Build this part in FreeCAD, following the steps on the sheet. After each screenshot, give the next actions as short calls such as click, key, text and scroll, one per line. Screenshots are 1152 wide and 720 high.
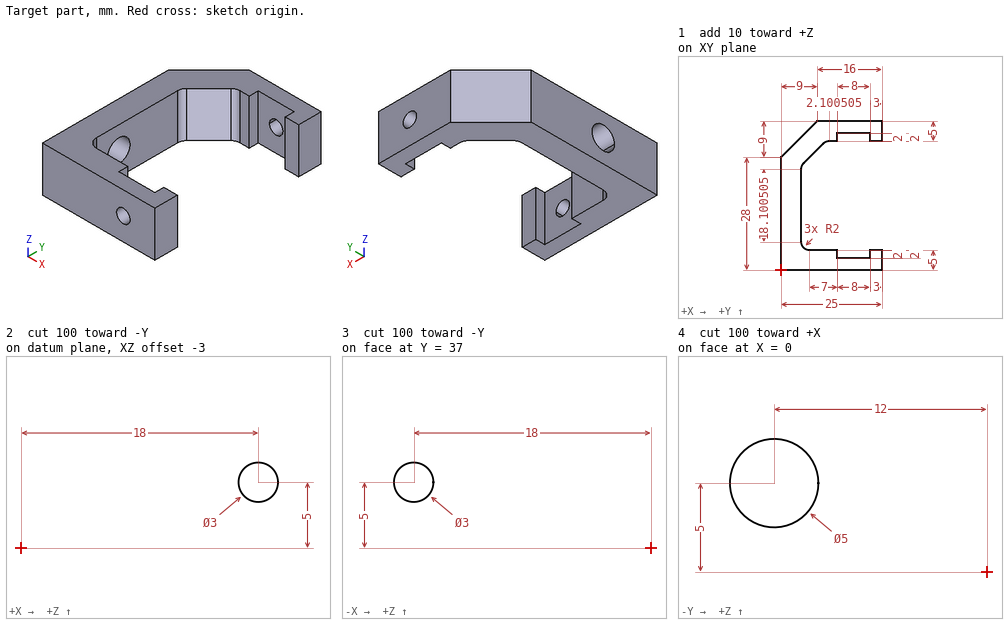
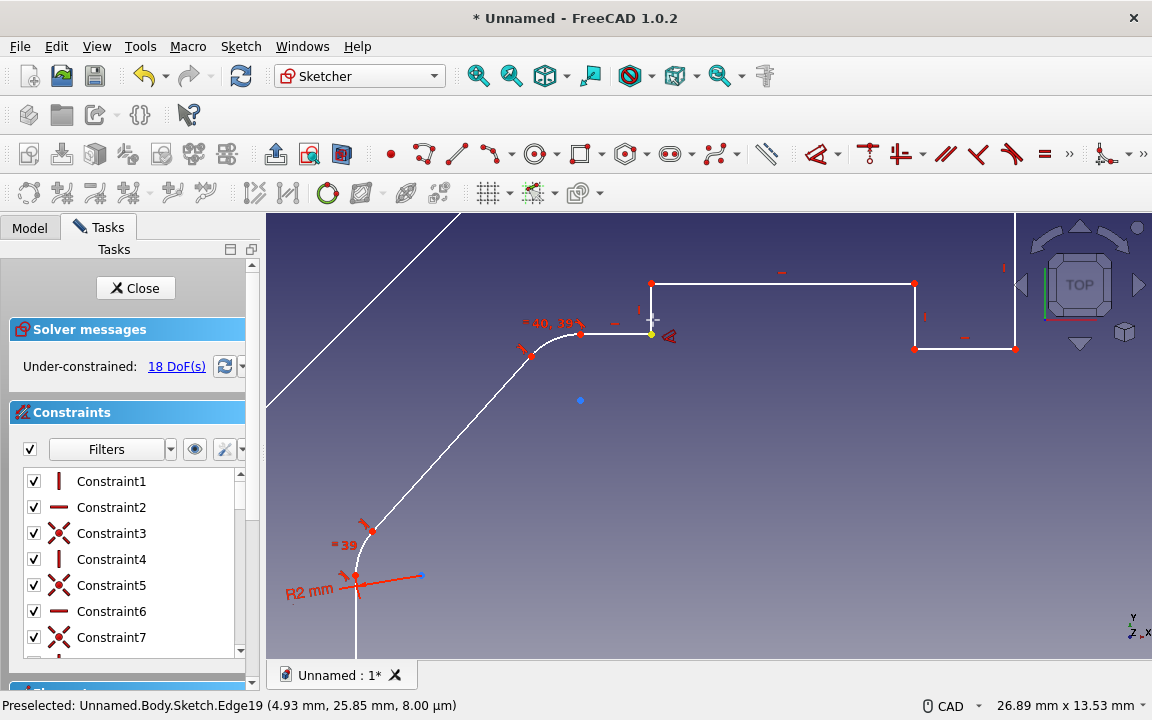
click(651, 319)
click(685, 309)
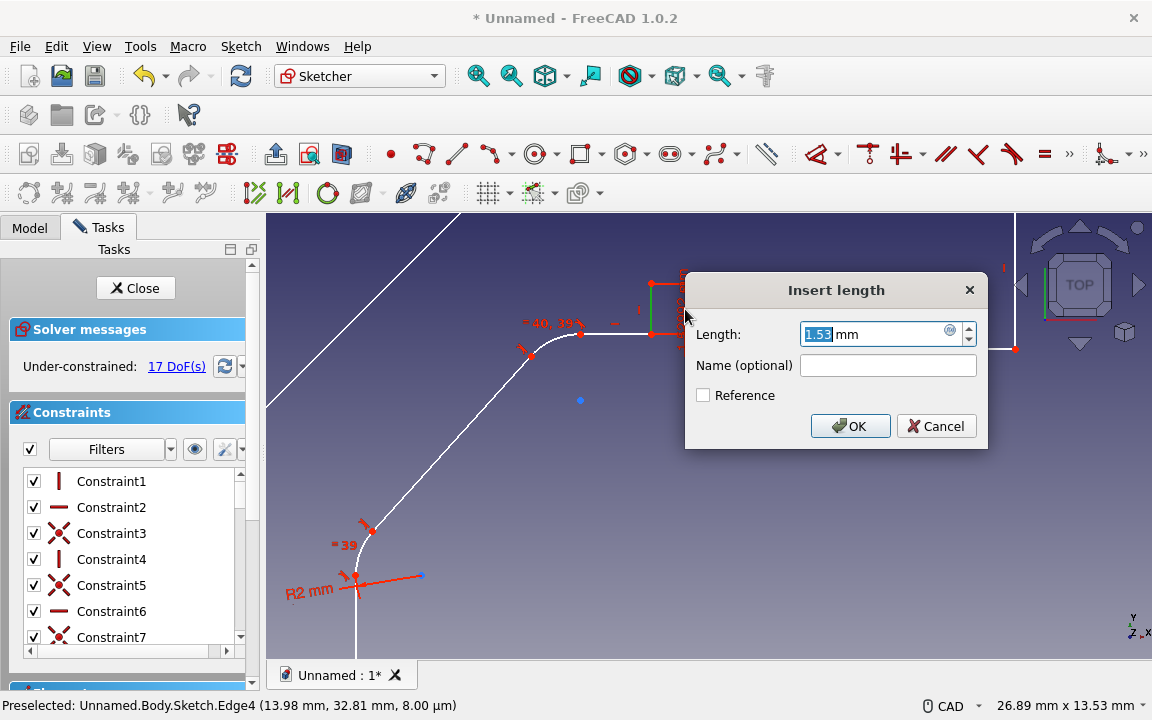
text(2)
key(Return)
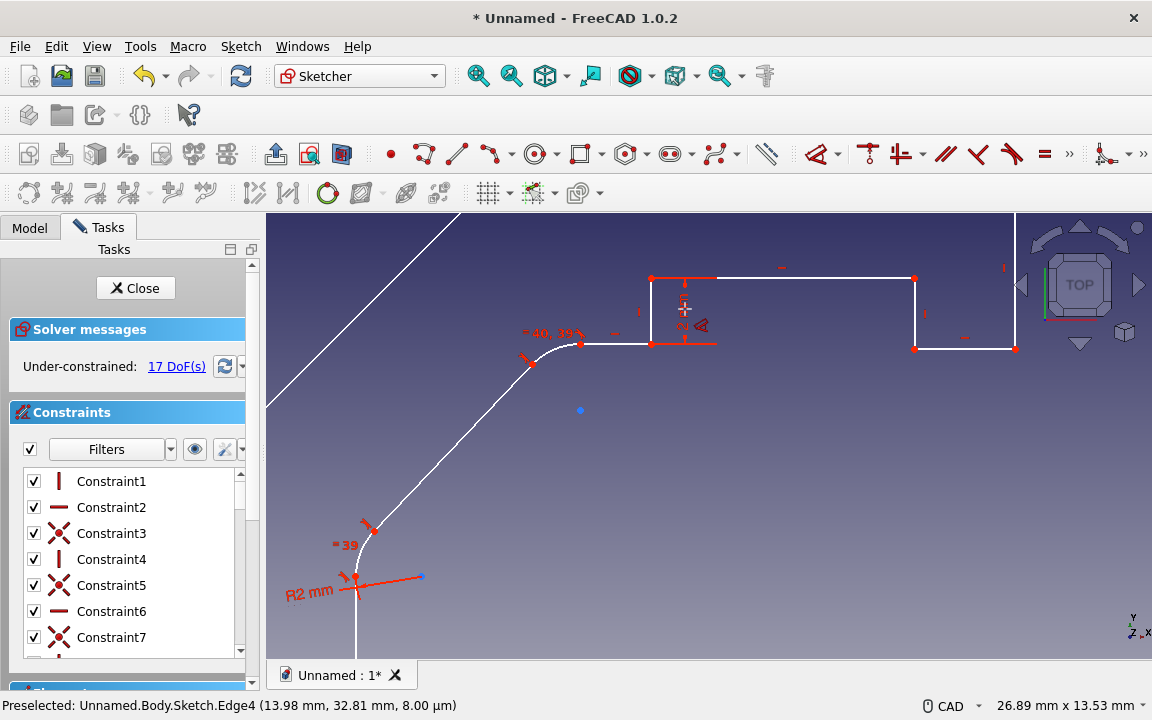
scroll(653, 320, down, 7)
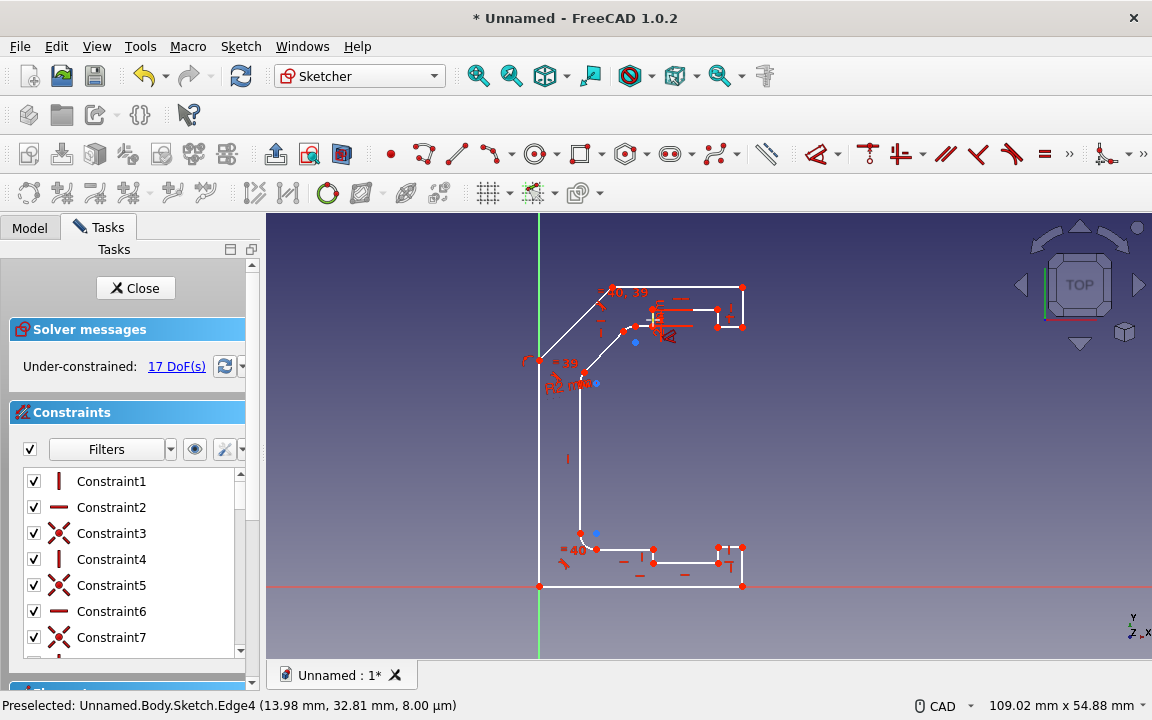
click(672, 310)
click(685, 344)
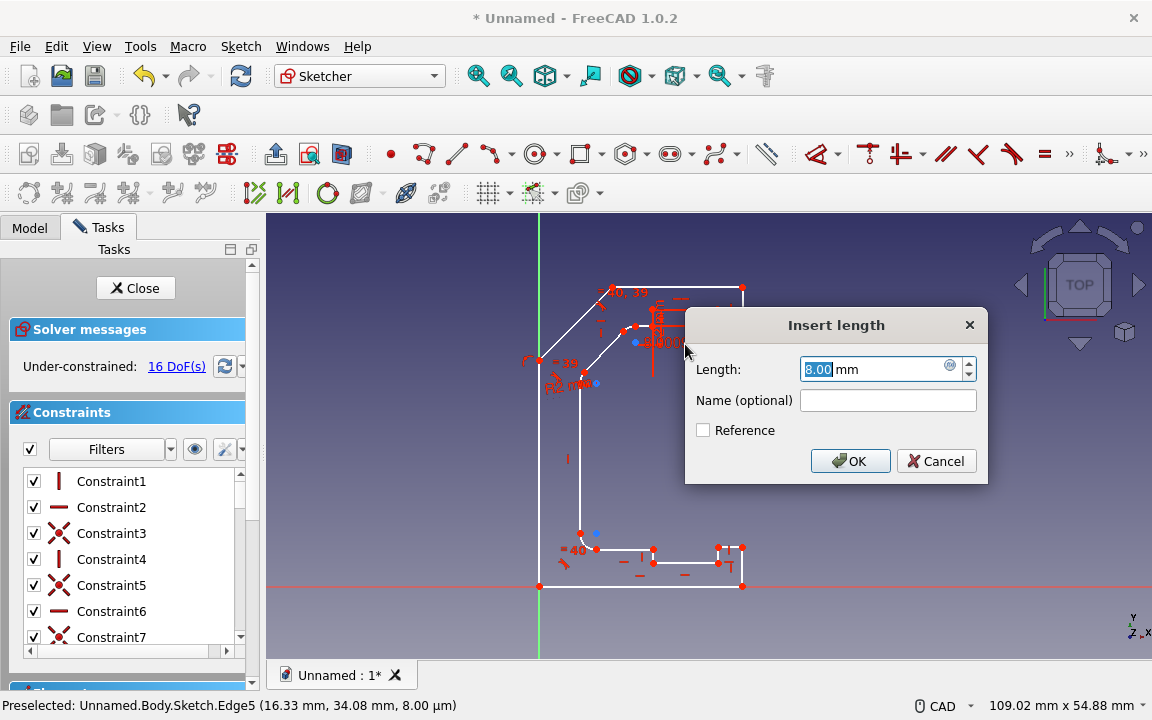
text(8)
key(Return)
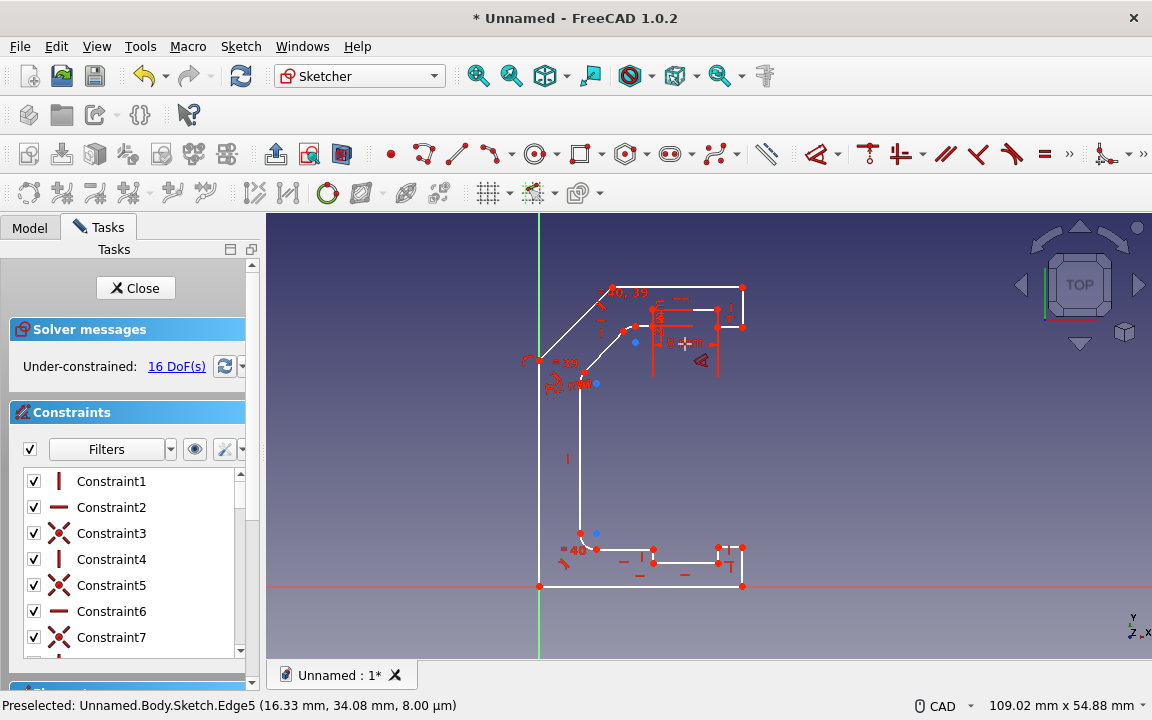
scroll(718, 319, up, 5)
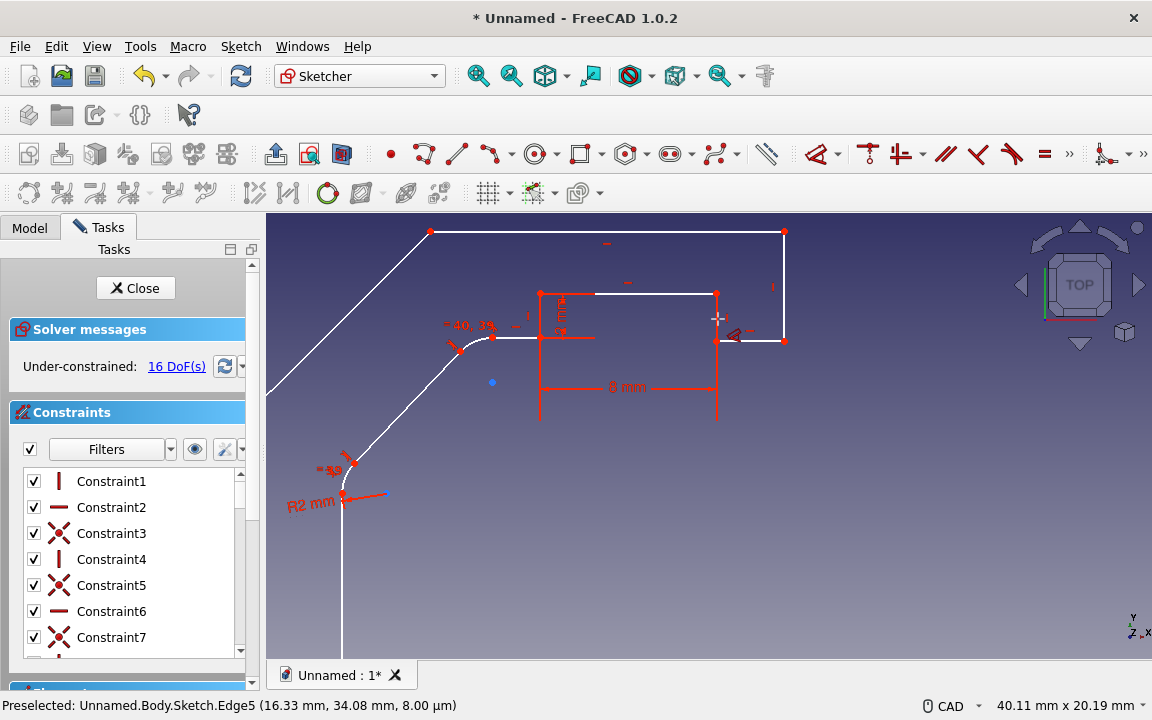
click(717, 318)
click(751, 318)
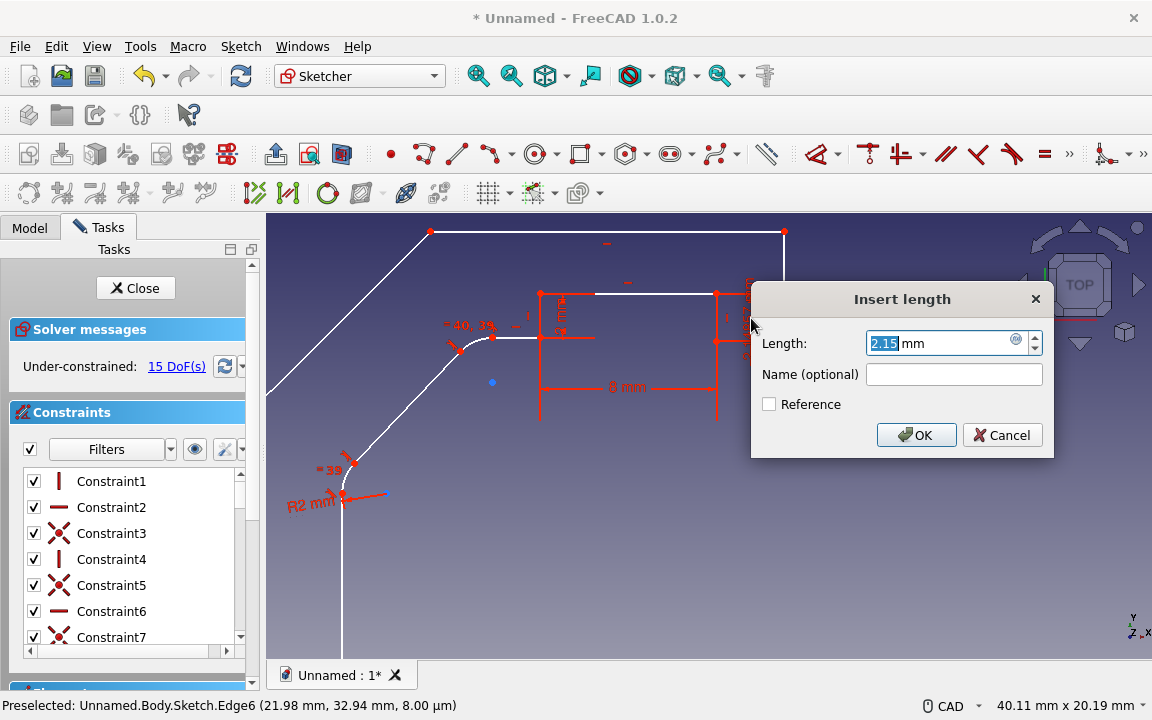
text(2)
key(Return)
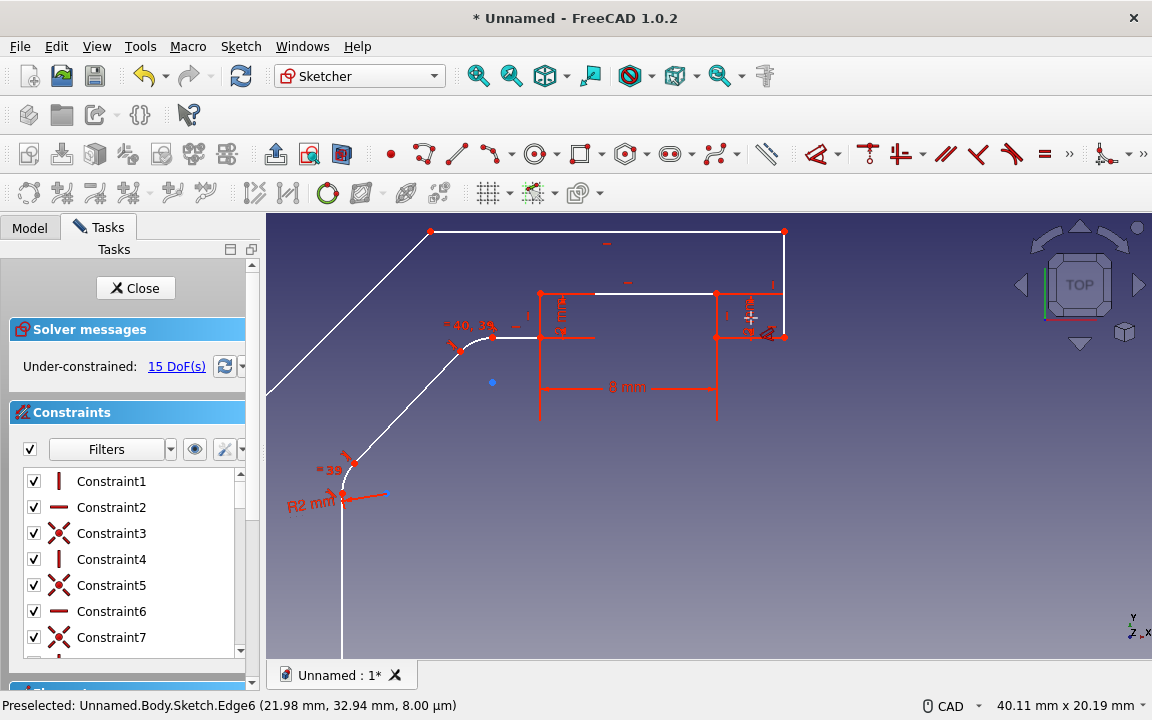
click(737, 338)
click(751, 372)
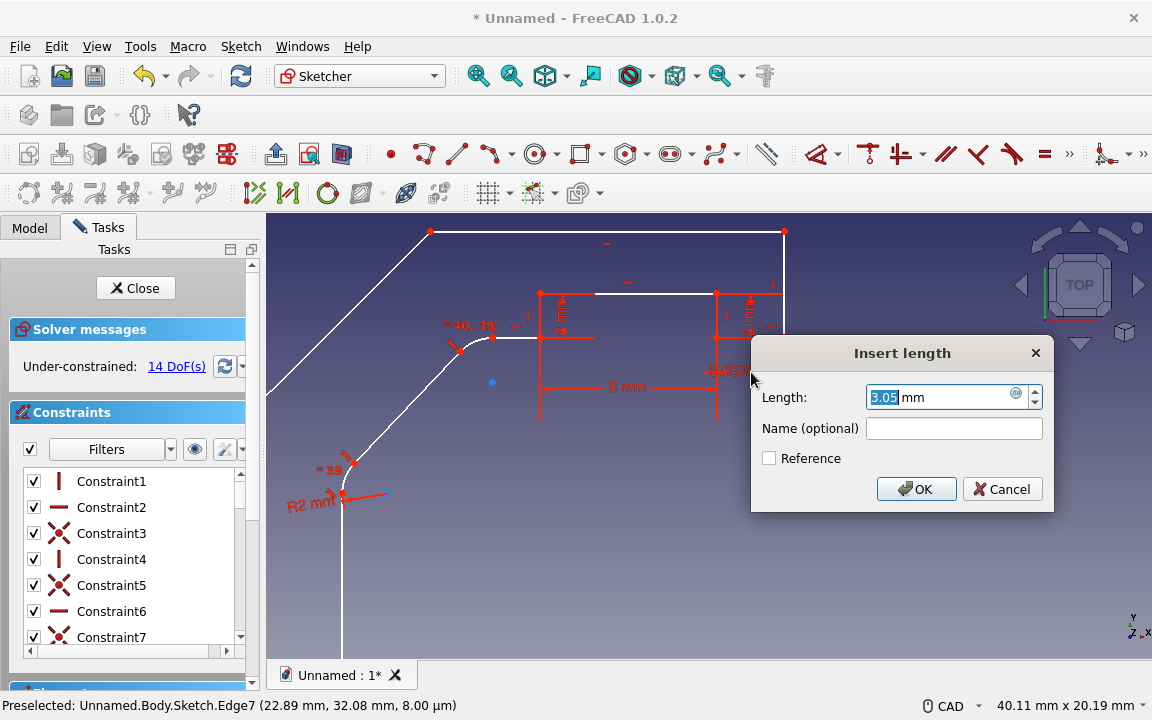
text(3)
key(Return)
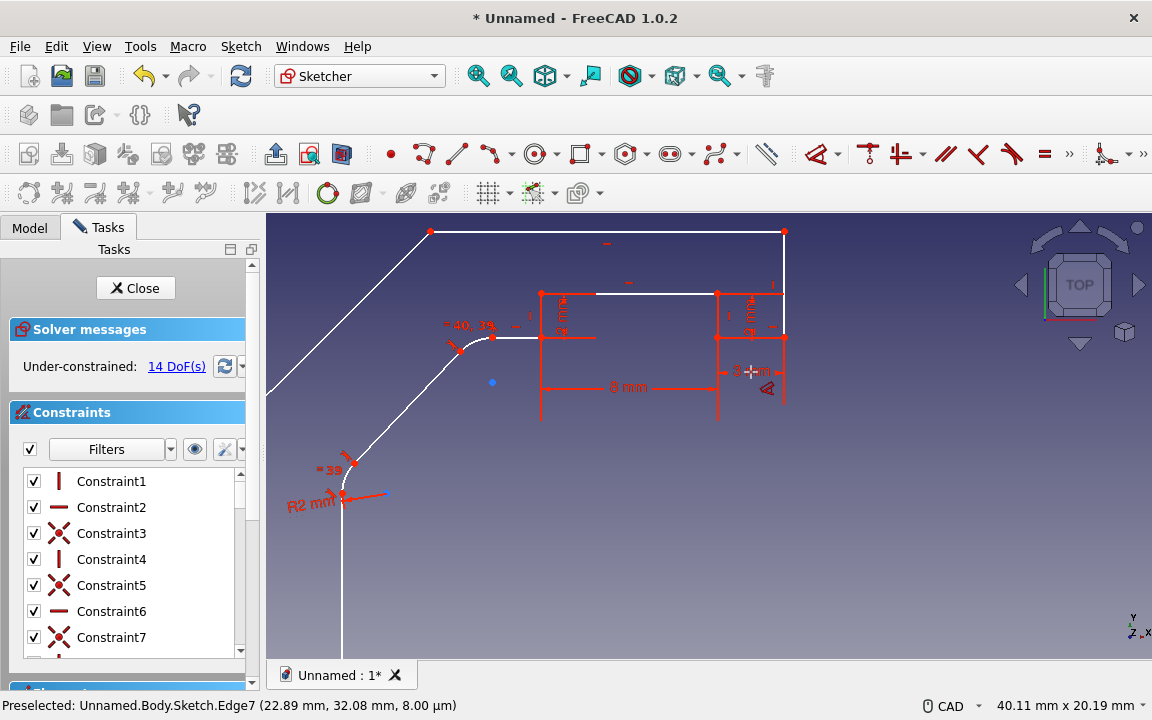
click(784, 306)
click(818, 289)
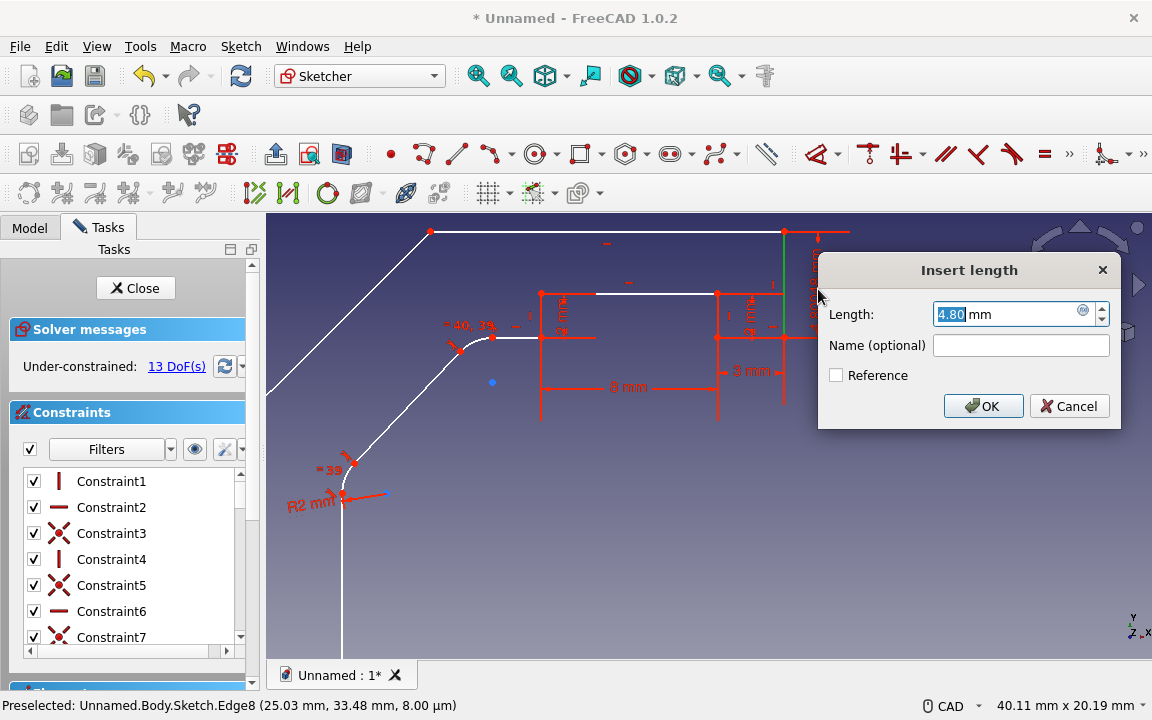
text(5)
key(Return)